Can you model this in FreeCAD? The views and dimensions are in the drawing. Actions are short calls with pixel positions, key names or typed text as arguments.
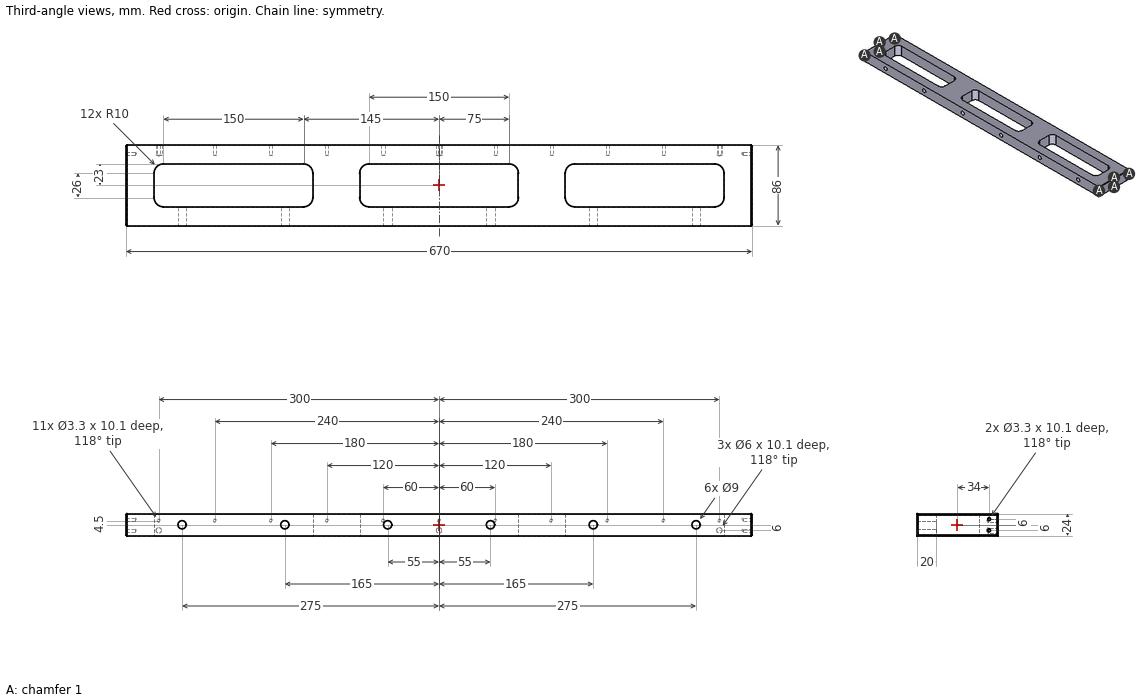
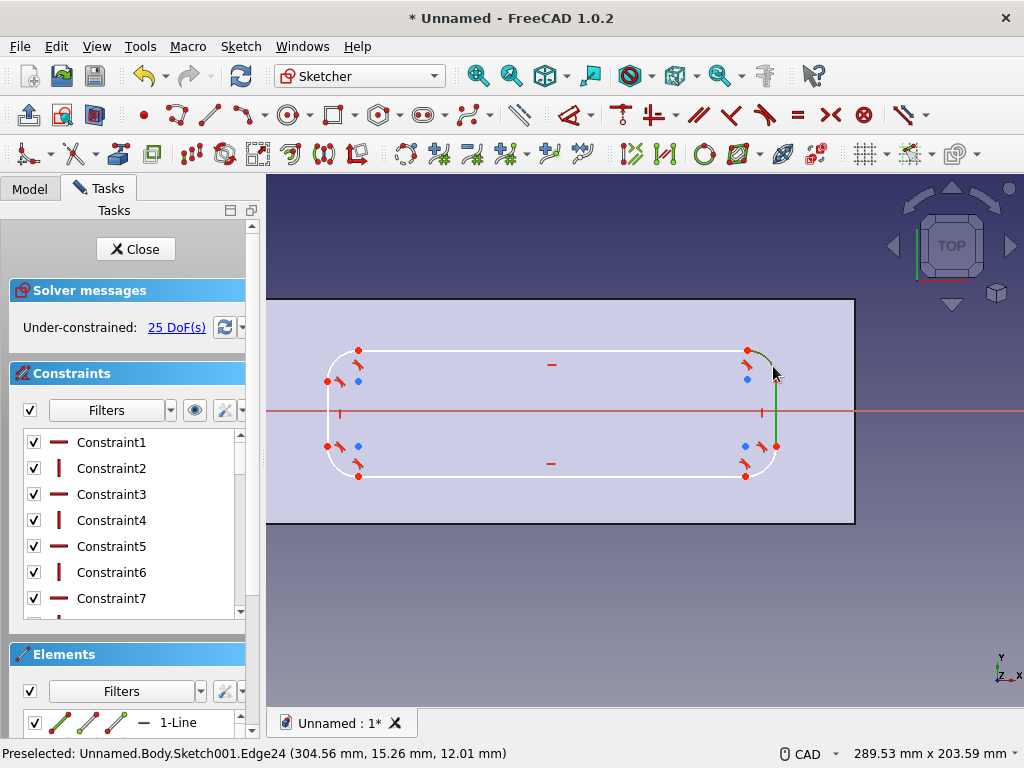
key(t)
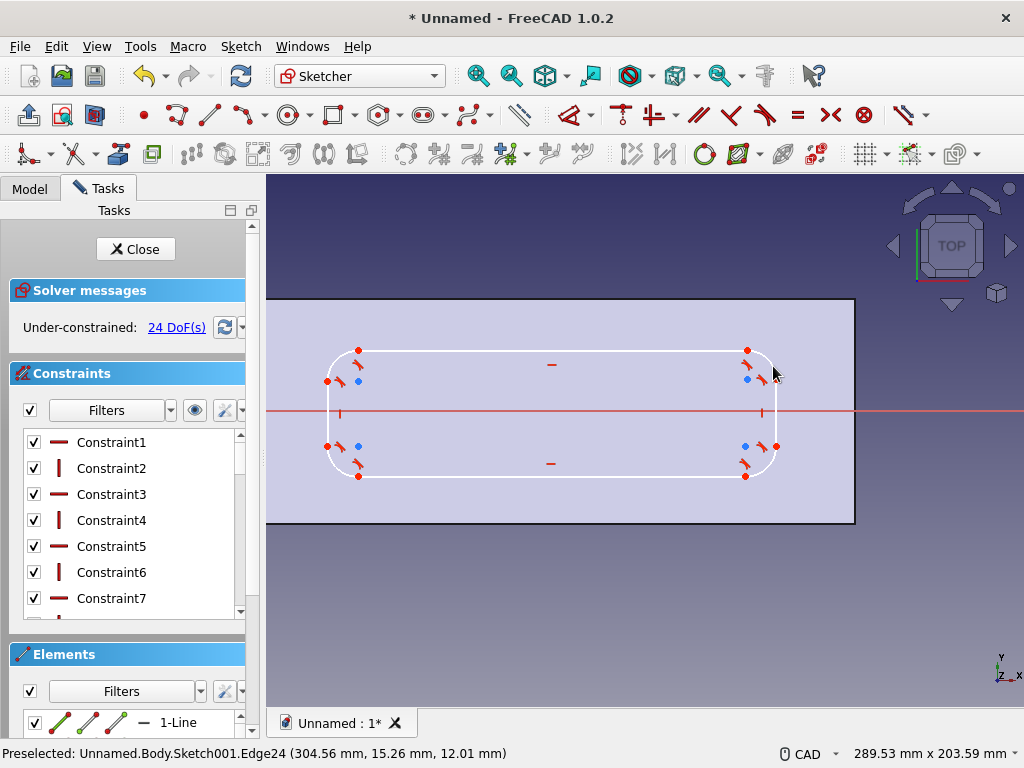
scroll(773, 450, down, 7)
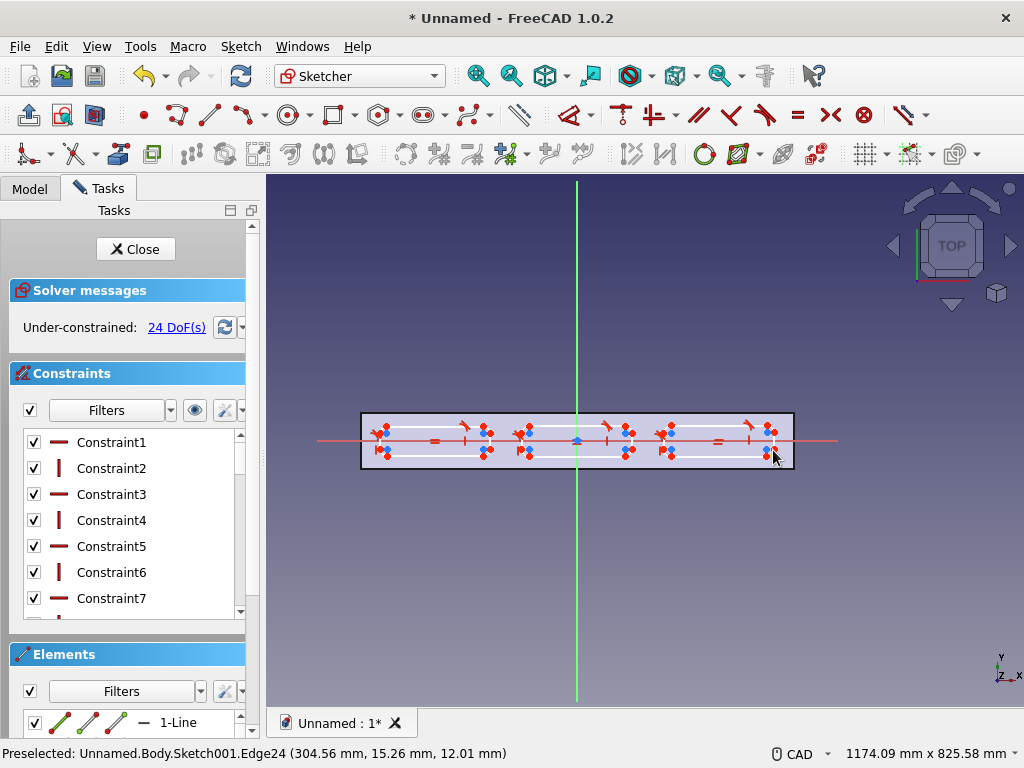
scroll(384, 427, up, 8)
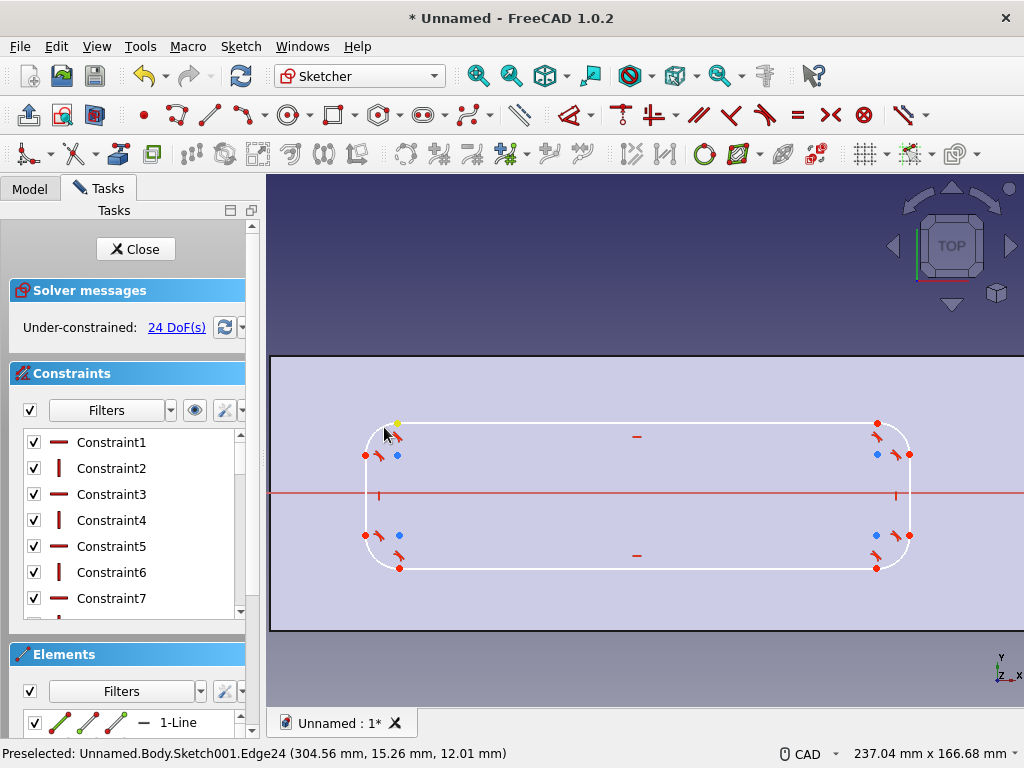
click(383, 427)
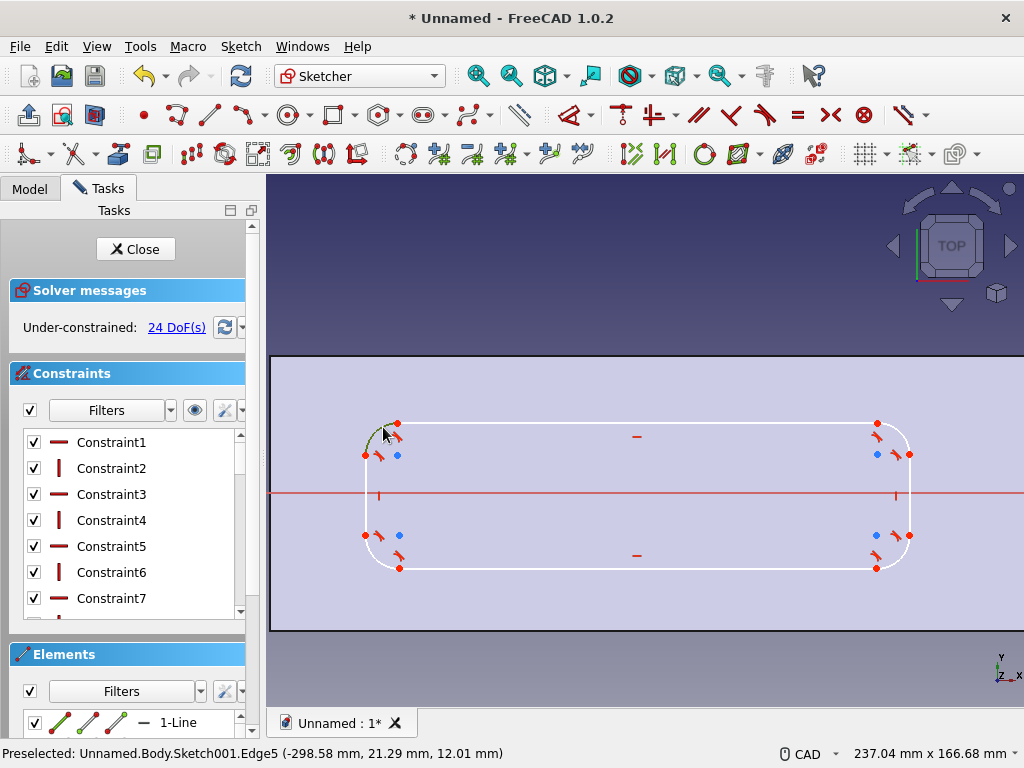
click(370, 551)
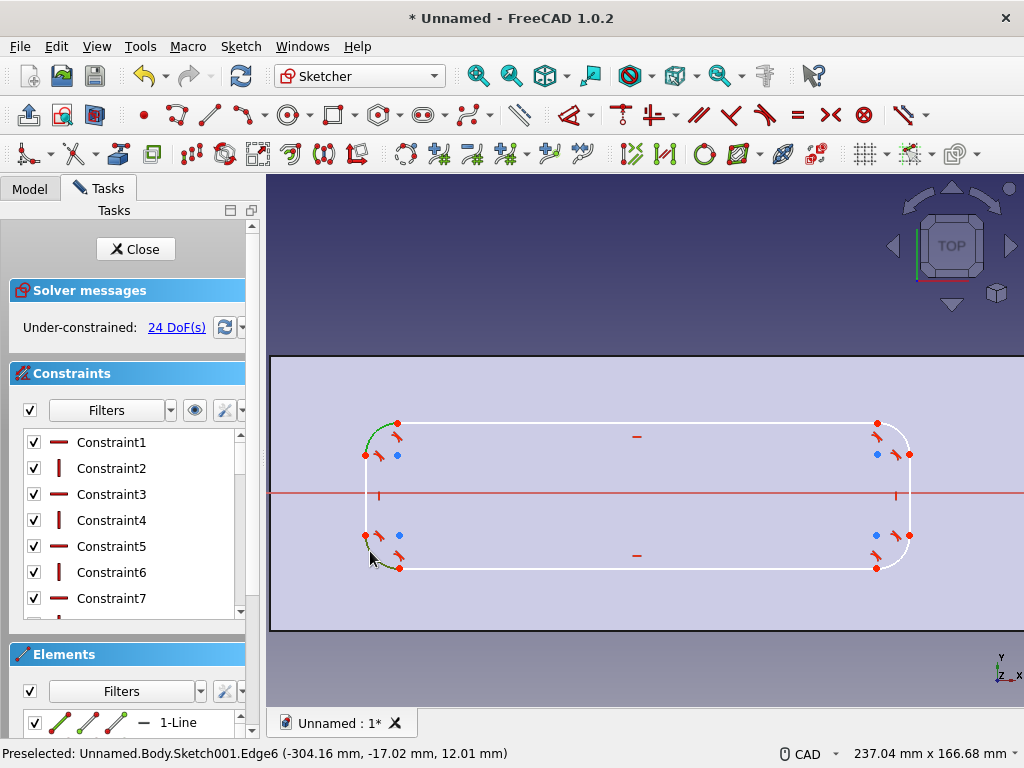
scroll(383, 427, down, 8)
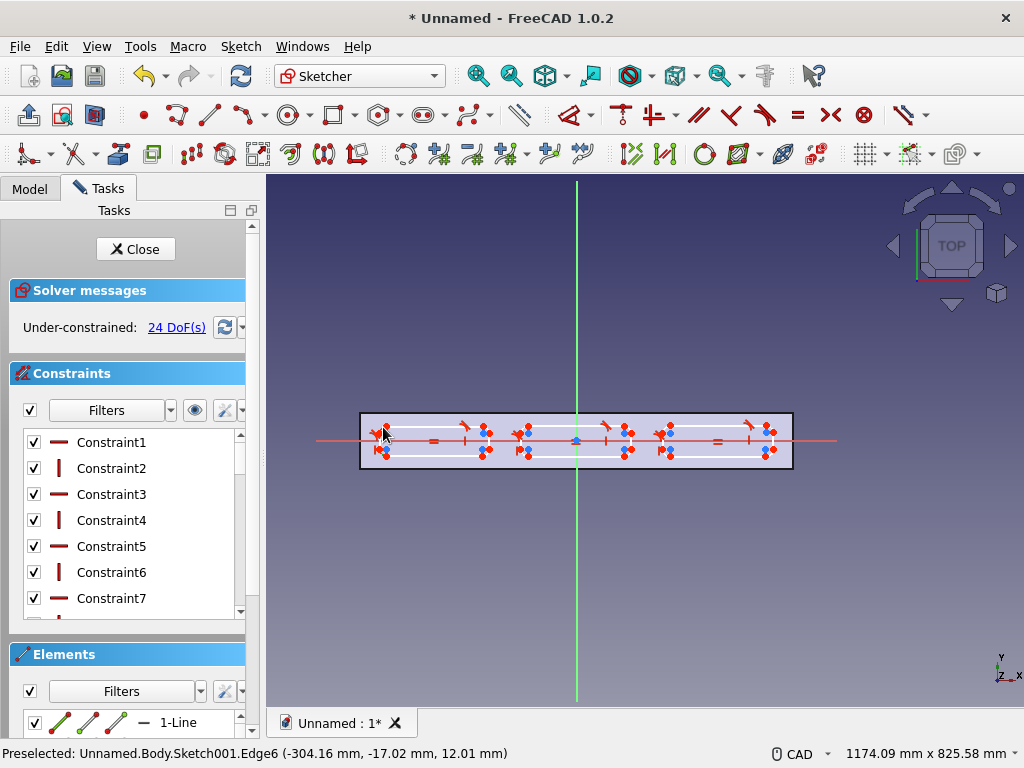
scroll(486, 455, up, 8)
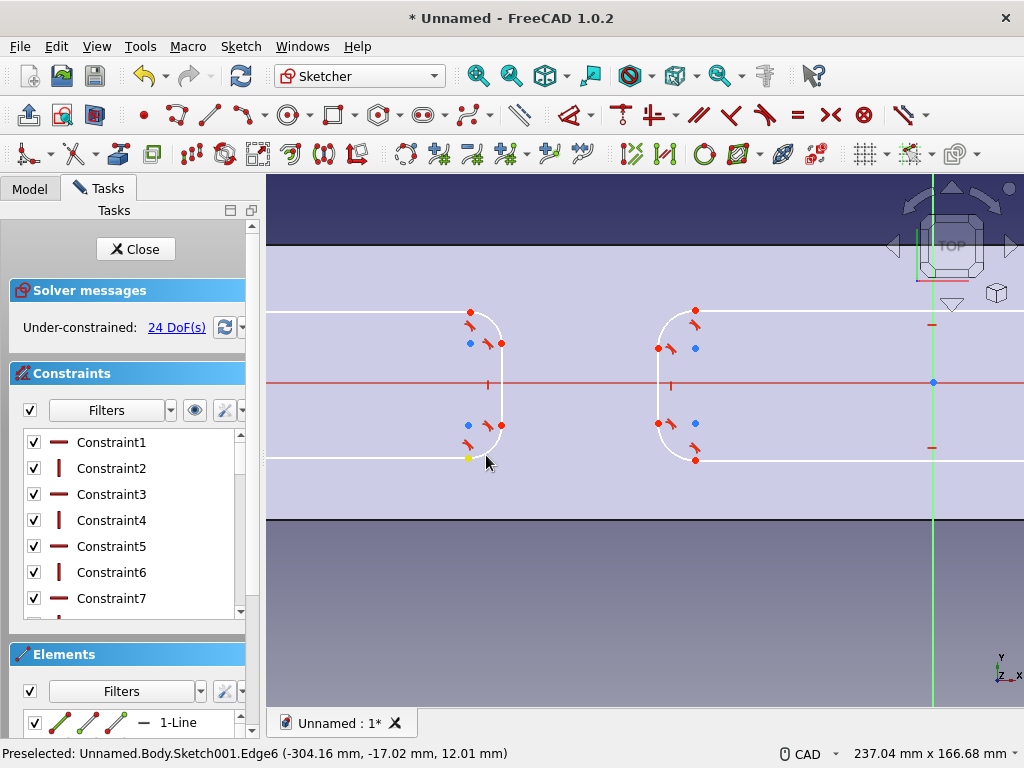
click(484, 455)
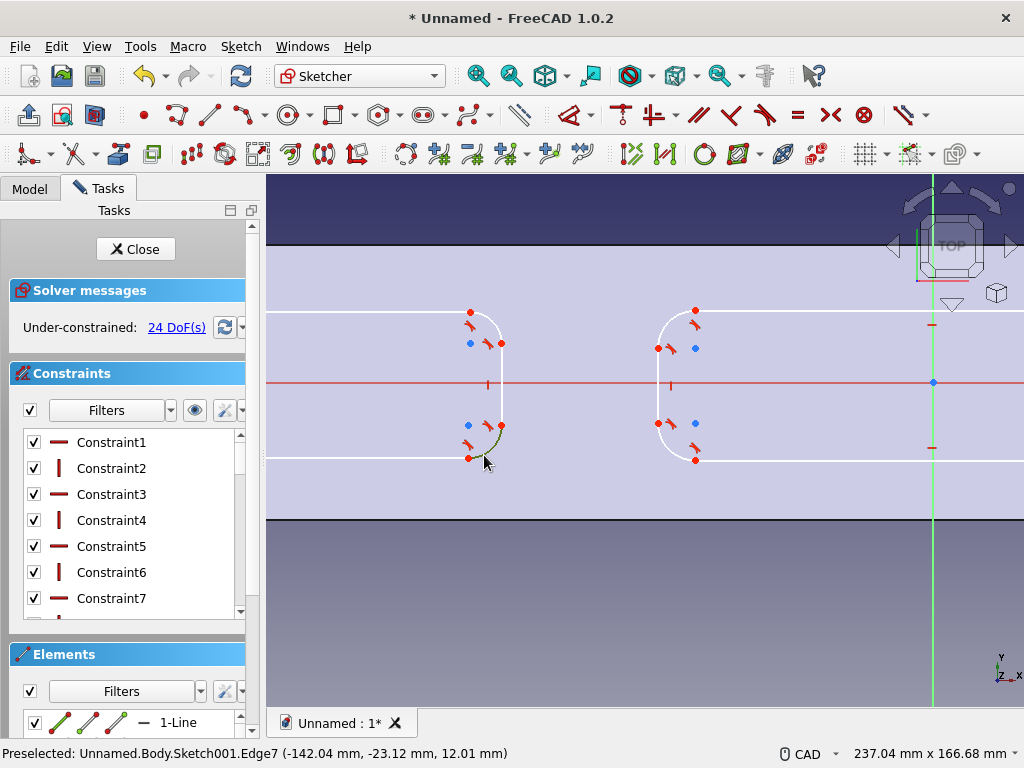
click(498, 330)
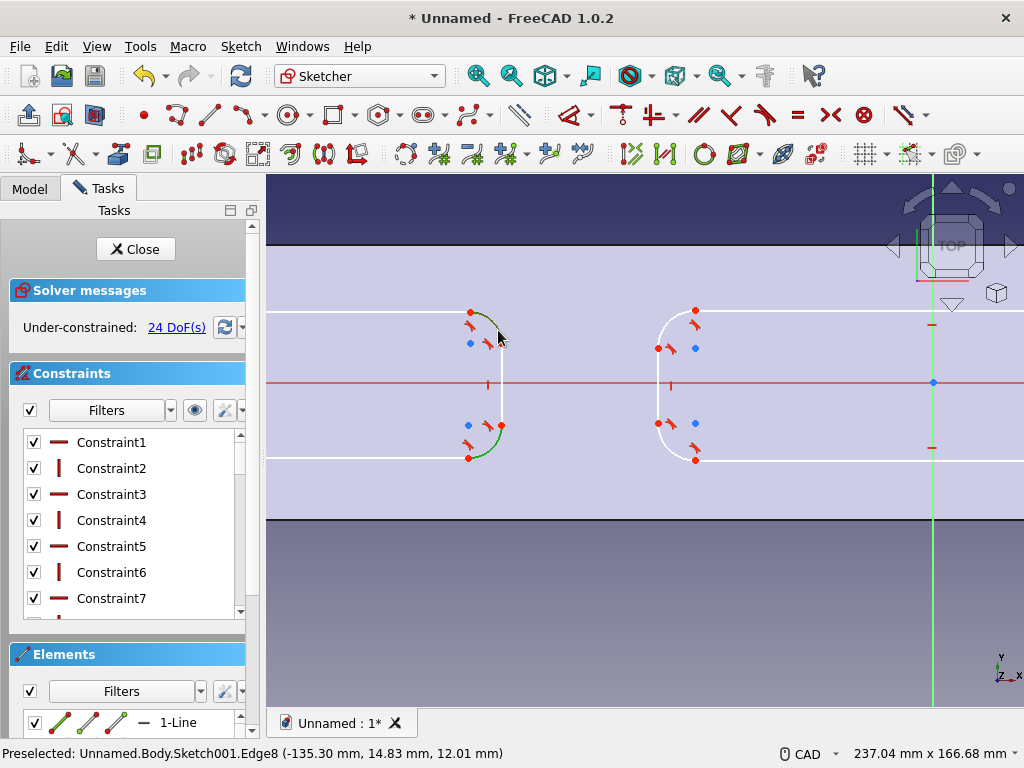
click(678, 315)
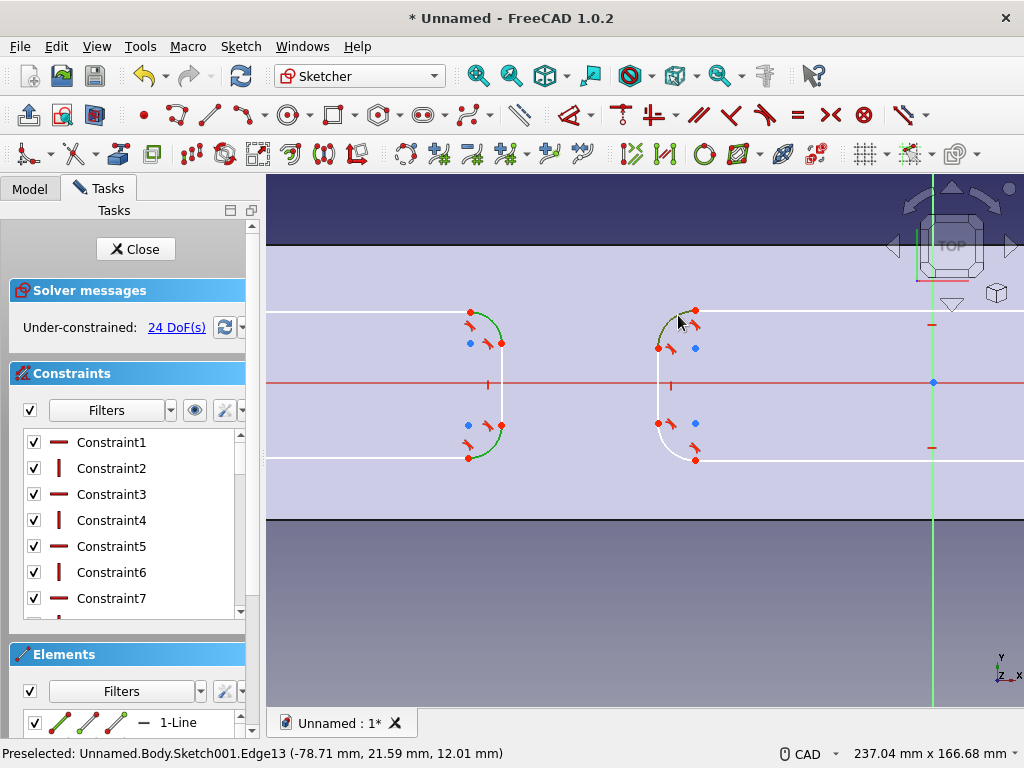
click(662, 440)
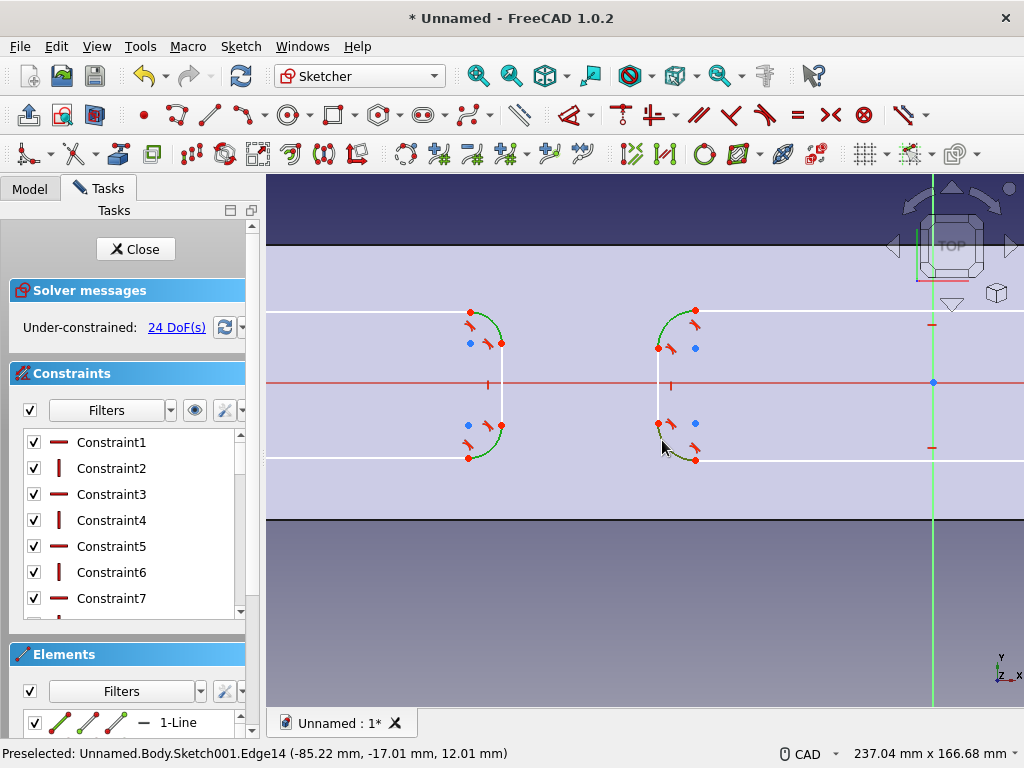
scroll(486, 455, down, 8)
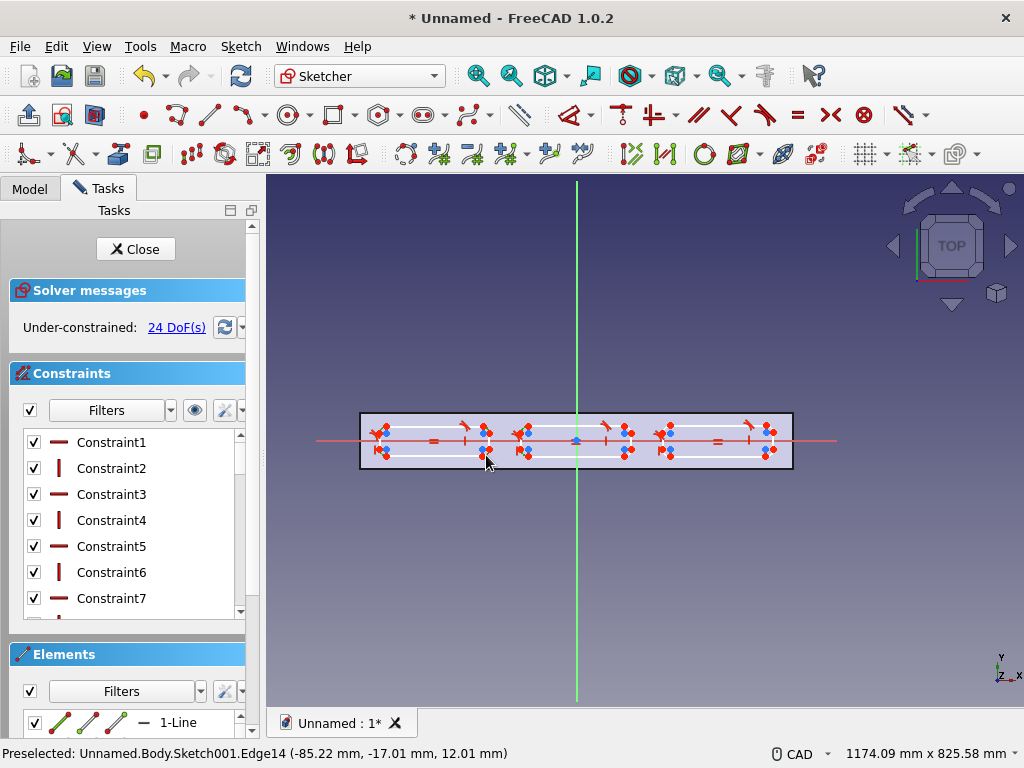
scroll(627, 456, up, 8)